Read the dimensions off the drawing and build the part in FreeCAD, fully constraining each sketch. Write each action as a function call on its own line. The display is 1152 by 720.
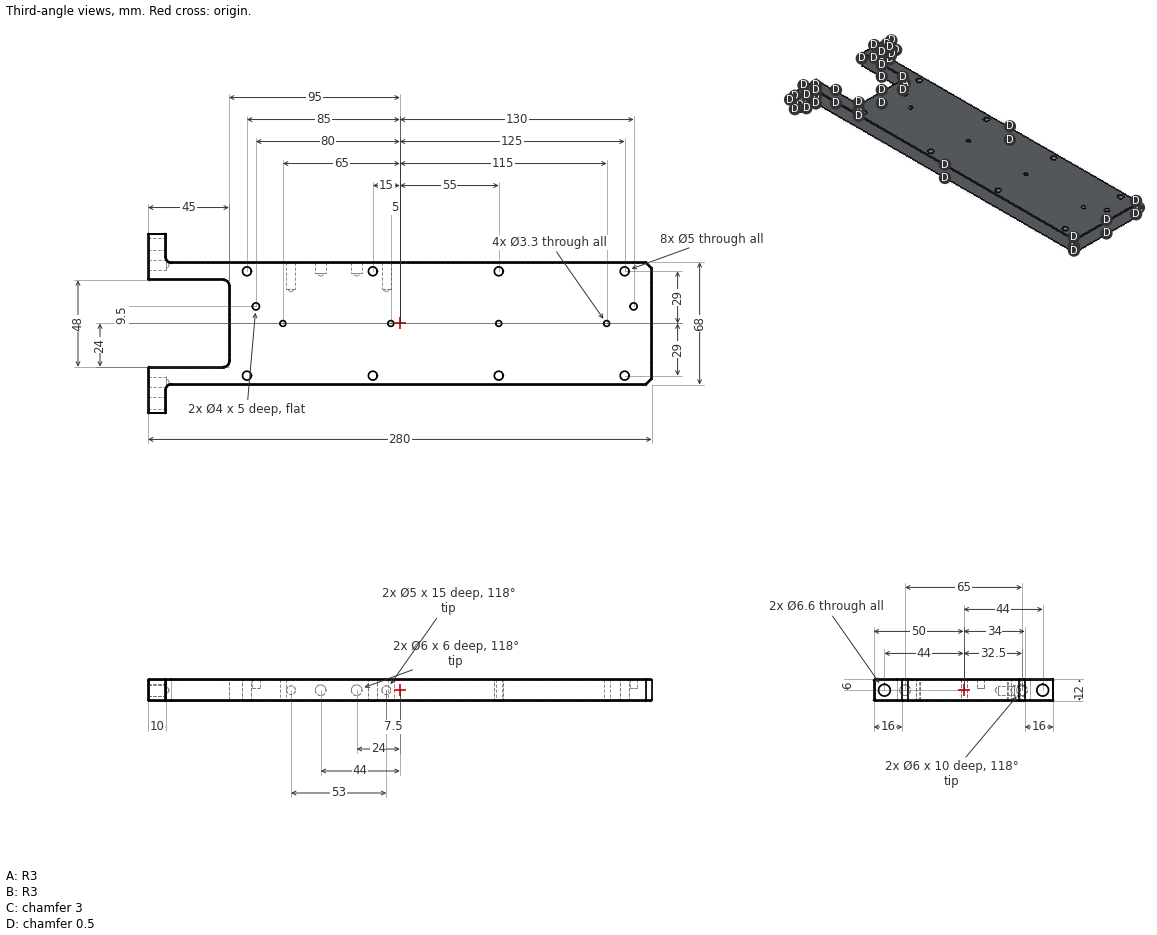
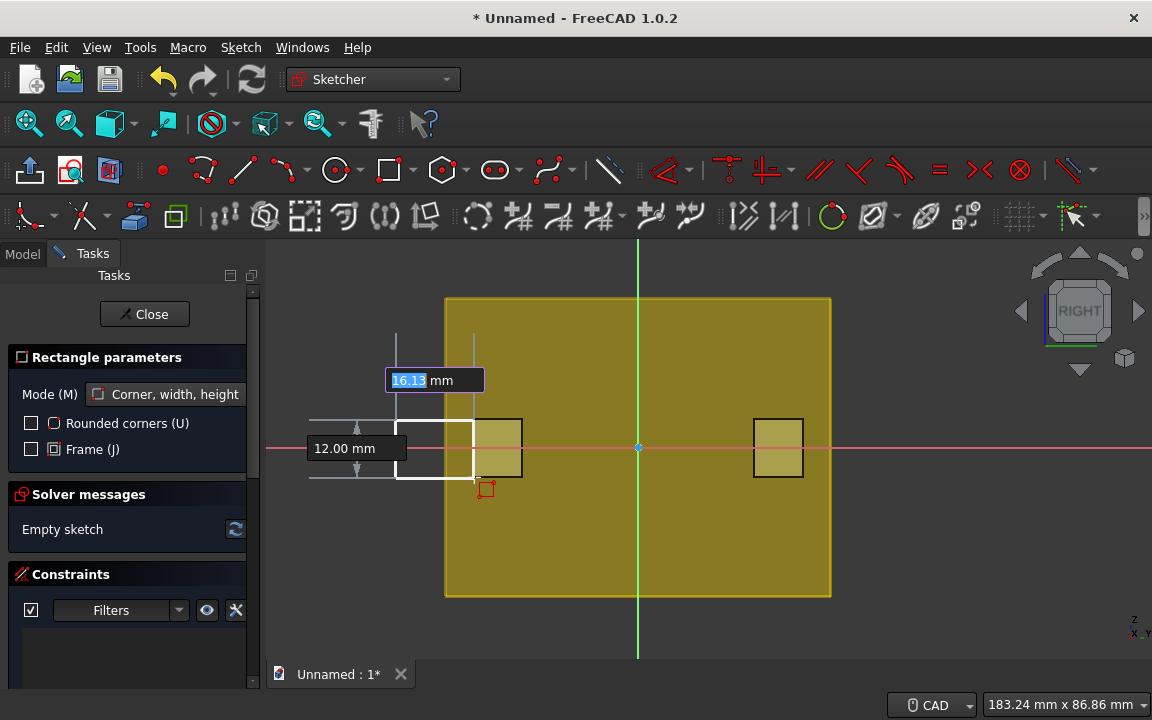
text(16)
key(Tab)
text(12)
key(Return)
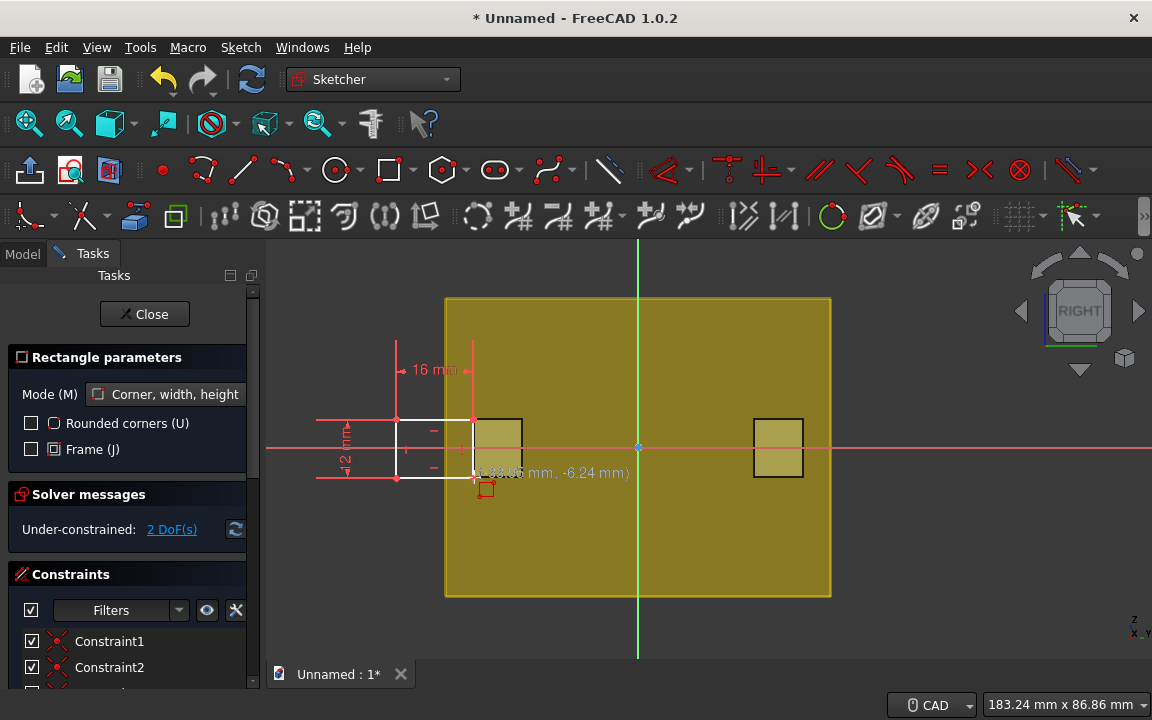
click(803, 419)
move(880, 477)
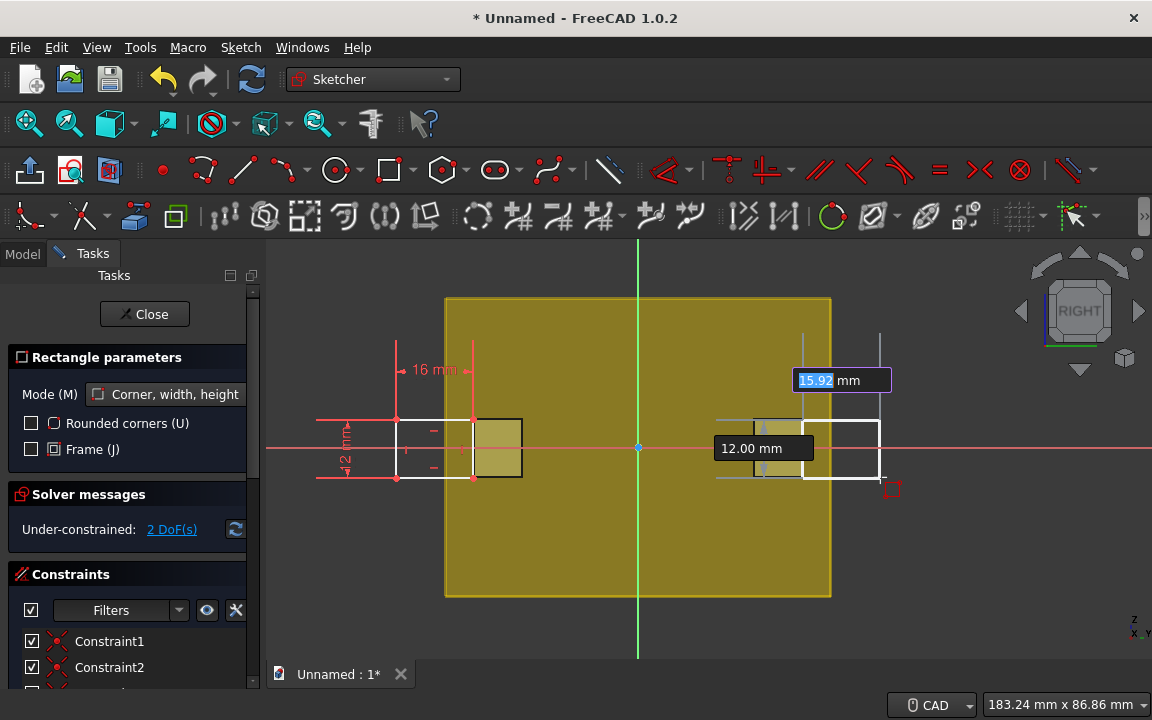
text(16)
key(Tab)
text(12)
key(Return)
key(Escape)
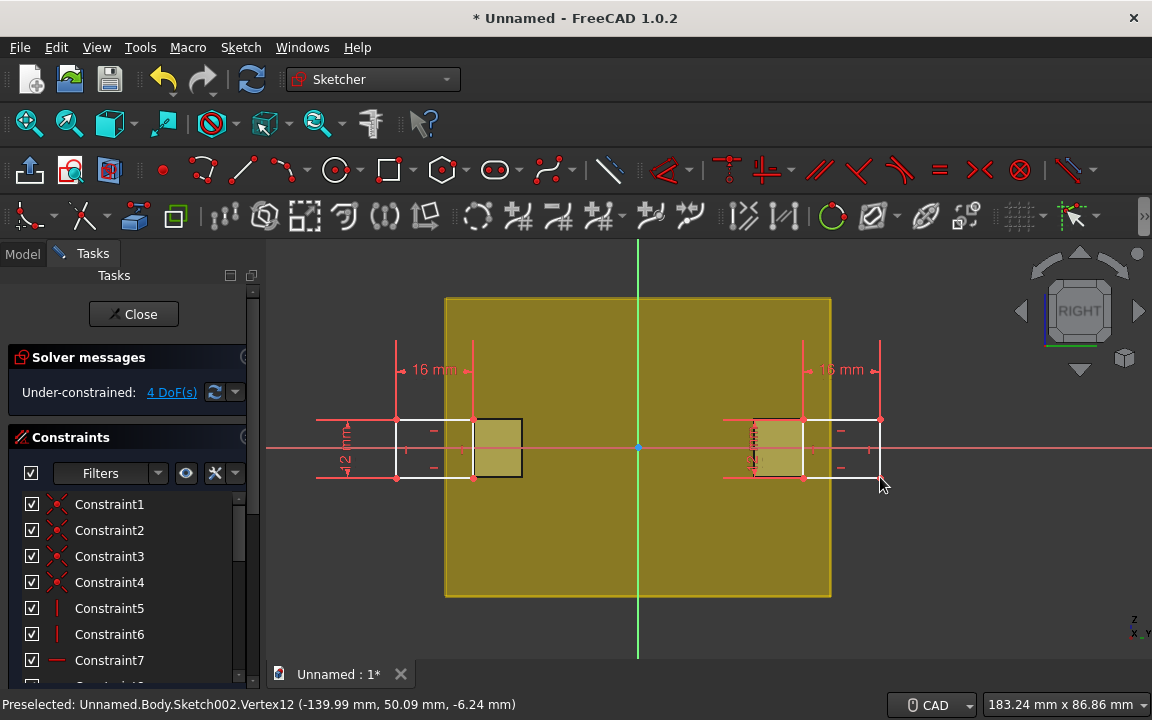
key(d)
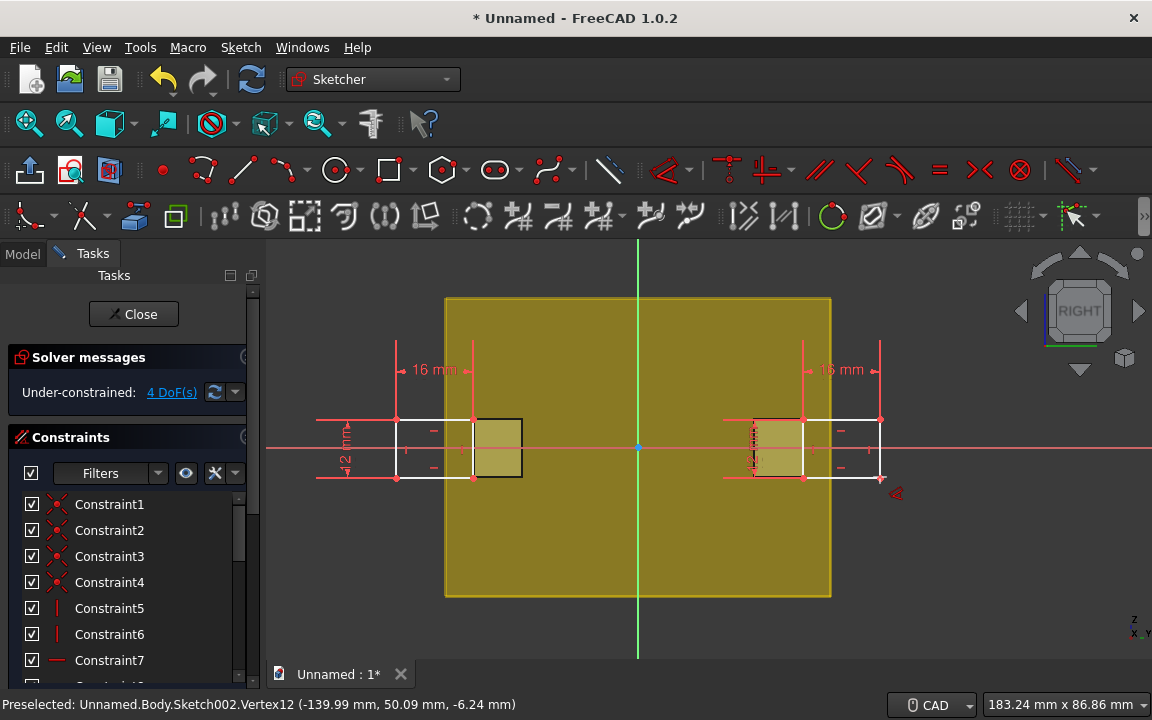
scroll(396, 420, up, 2)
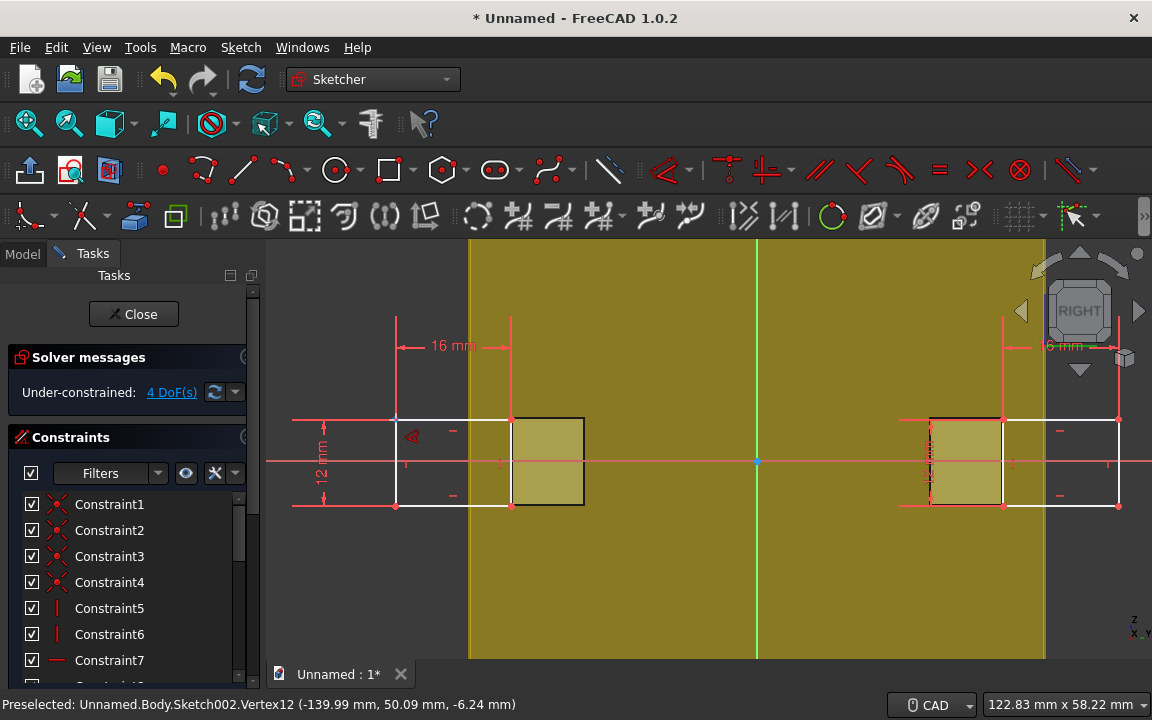
click(396, 420)
click(362, 441)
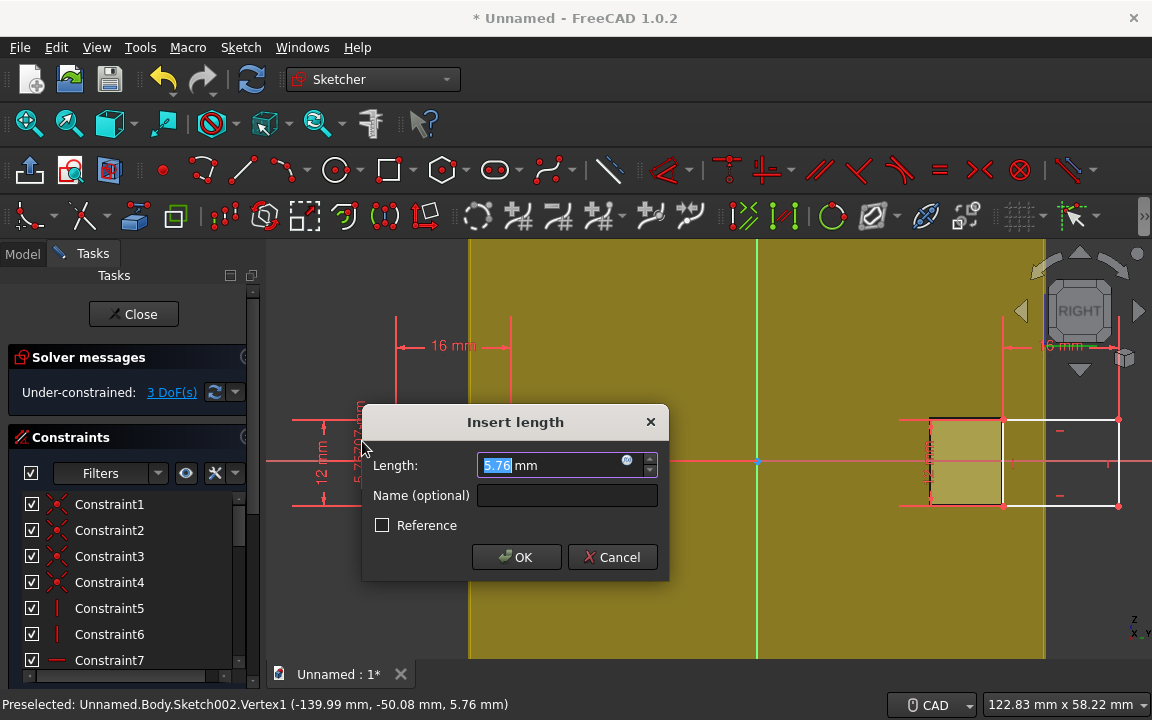
text(6)
key(Return)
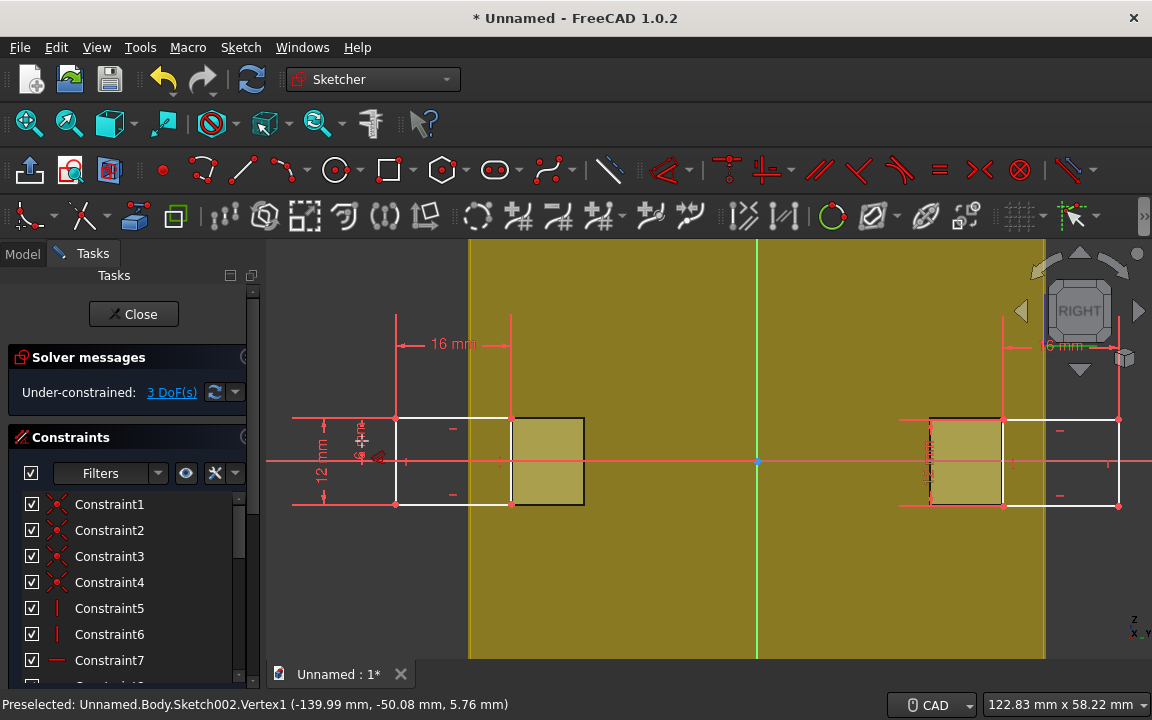
scroll(403, 424, down, 2)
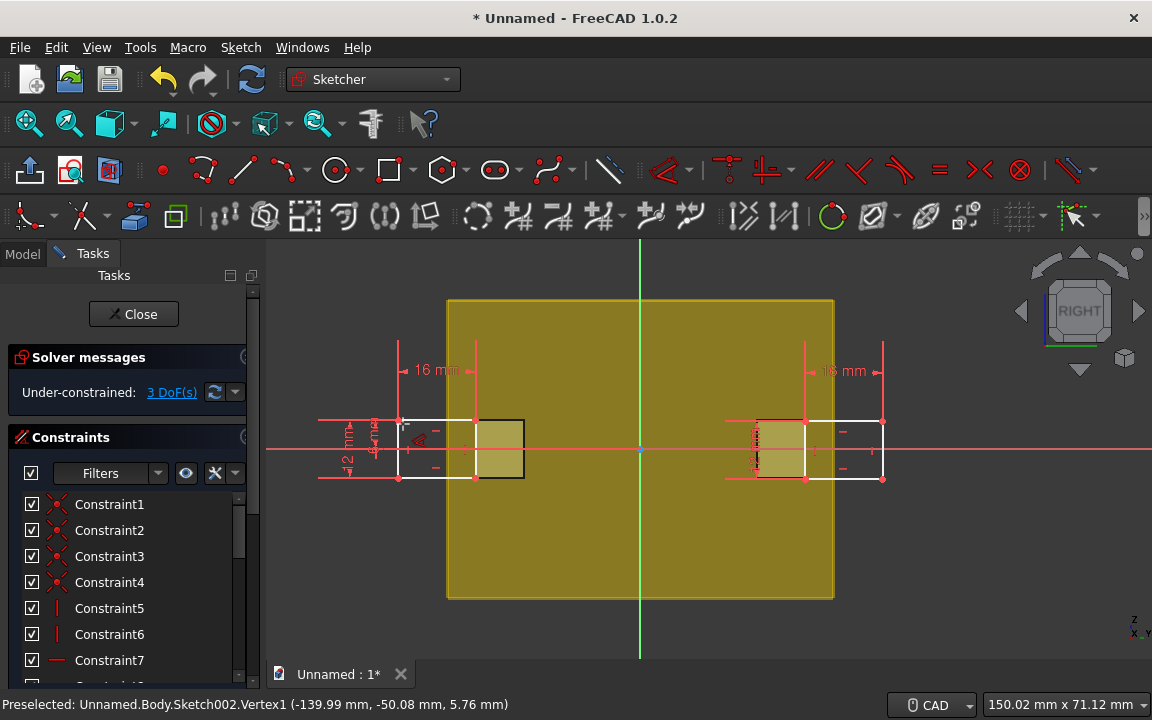
scroll(805, 421, up, 2)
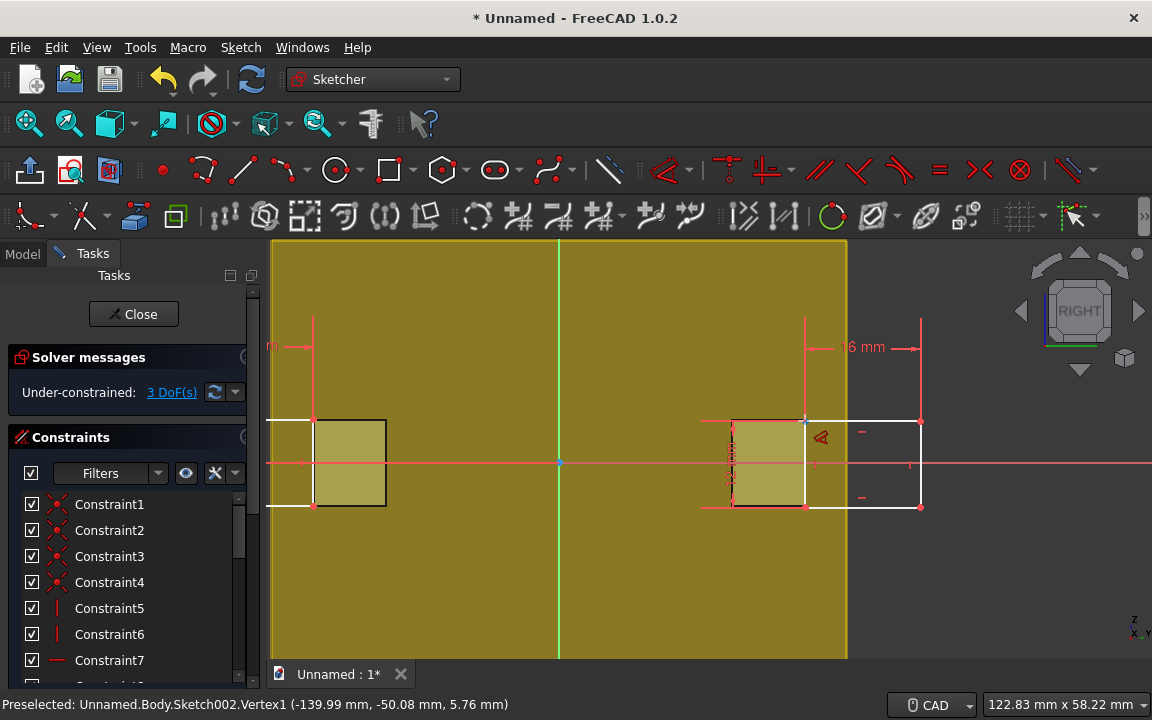
click(805, 421)
click(839, 442)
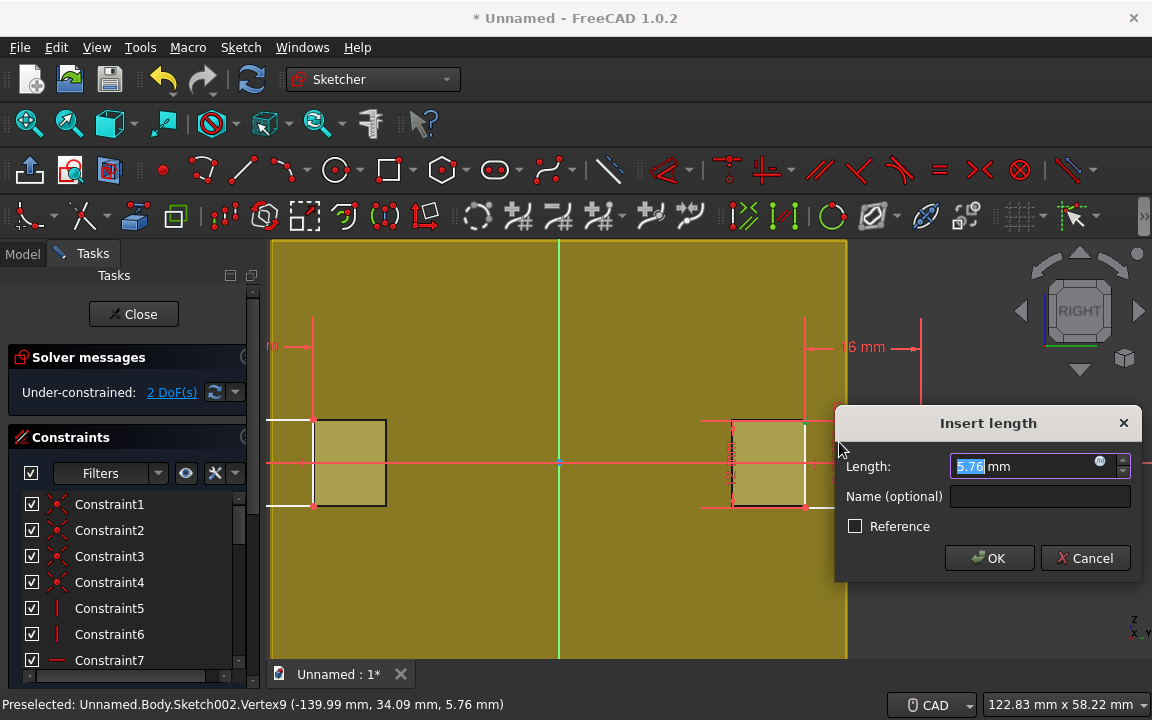
text(6)
key(Return)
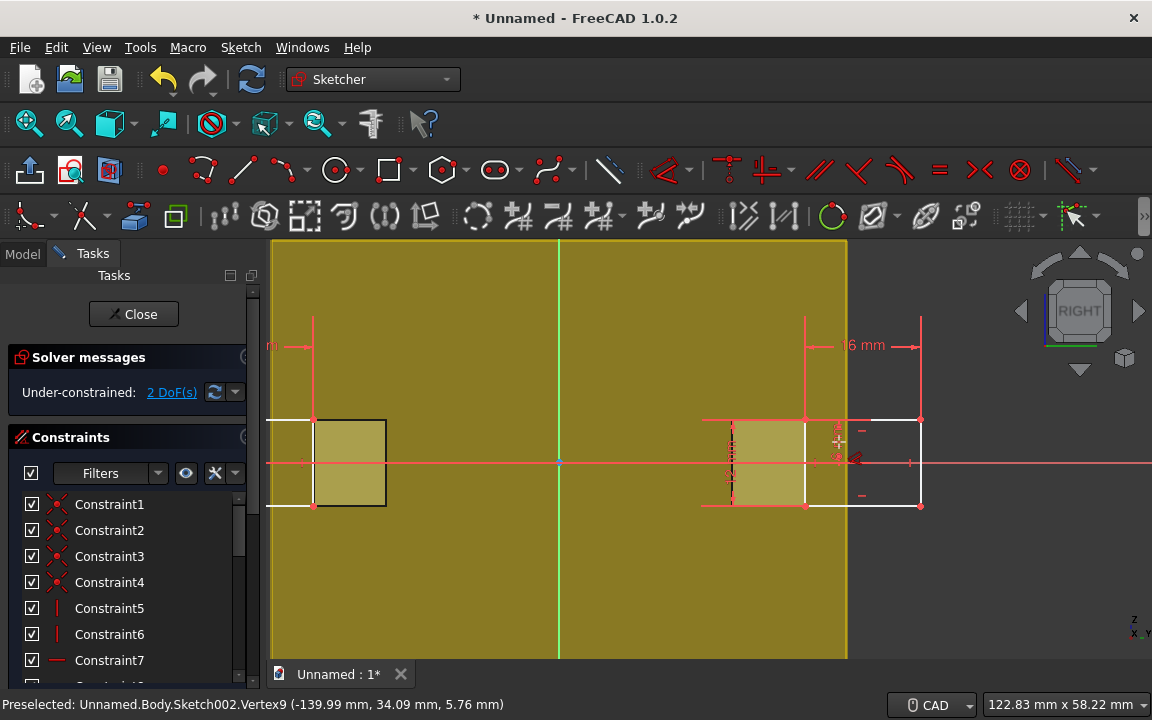
scroll(806, 421, down, 2)